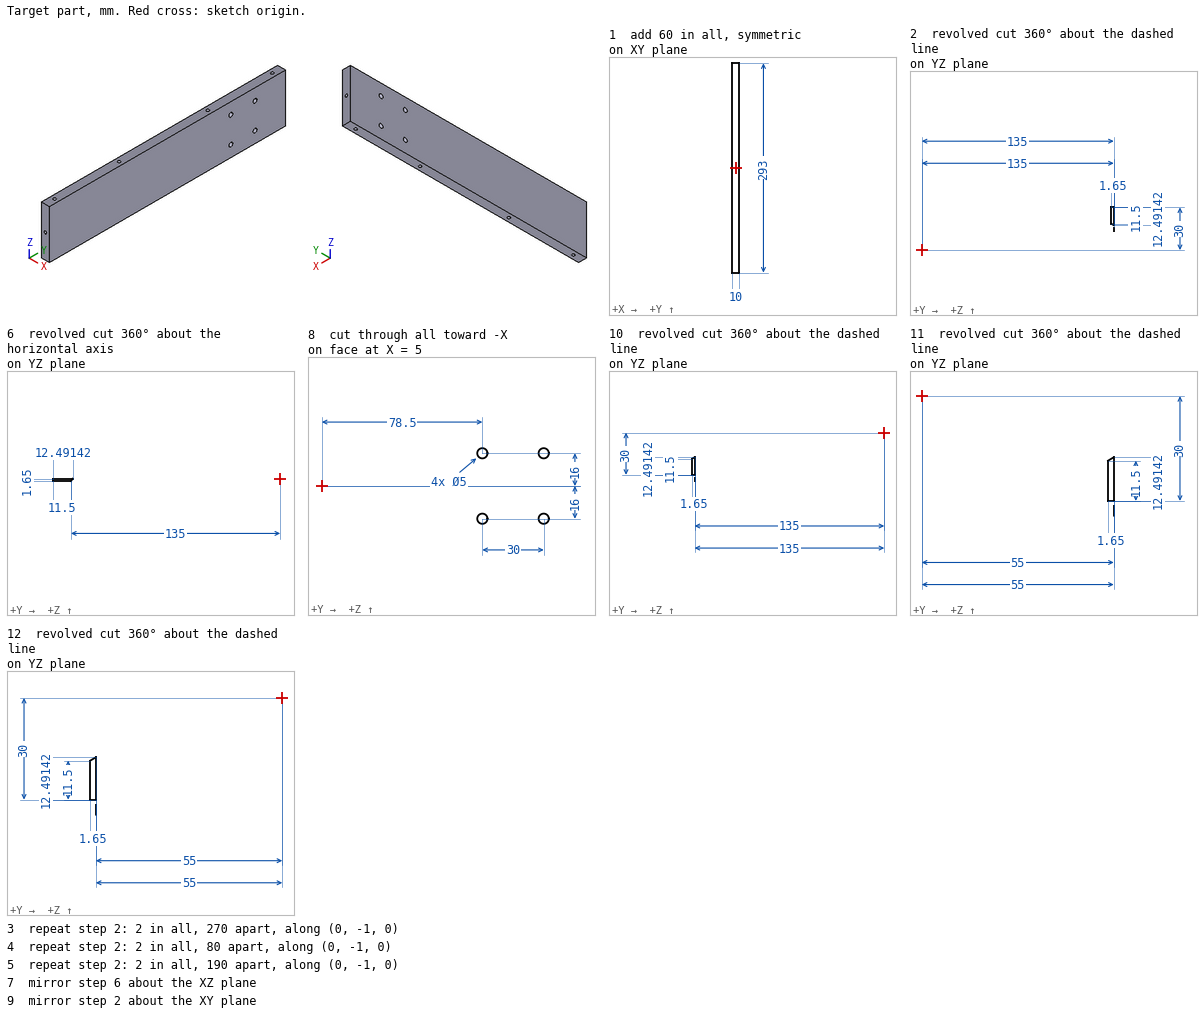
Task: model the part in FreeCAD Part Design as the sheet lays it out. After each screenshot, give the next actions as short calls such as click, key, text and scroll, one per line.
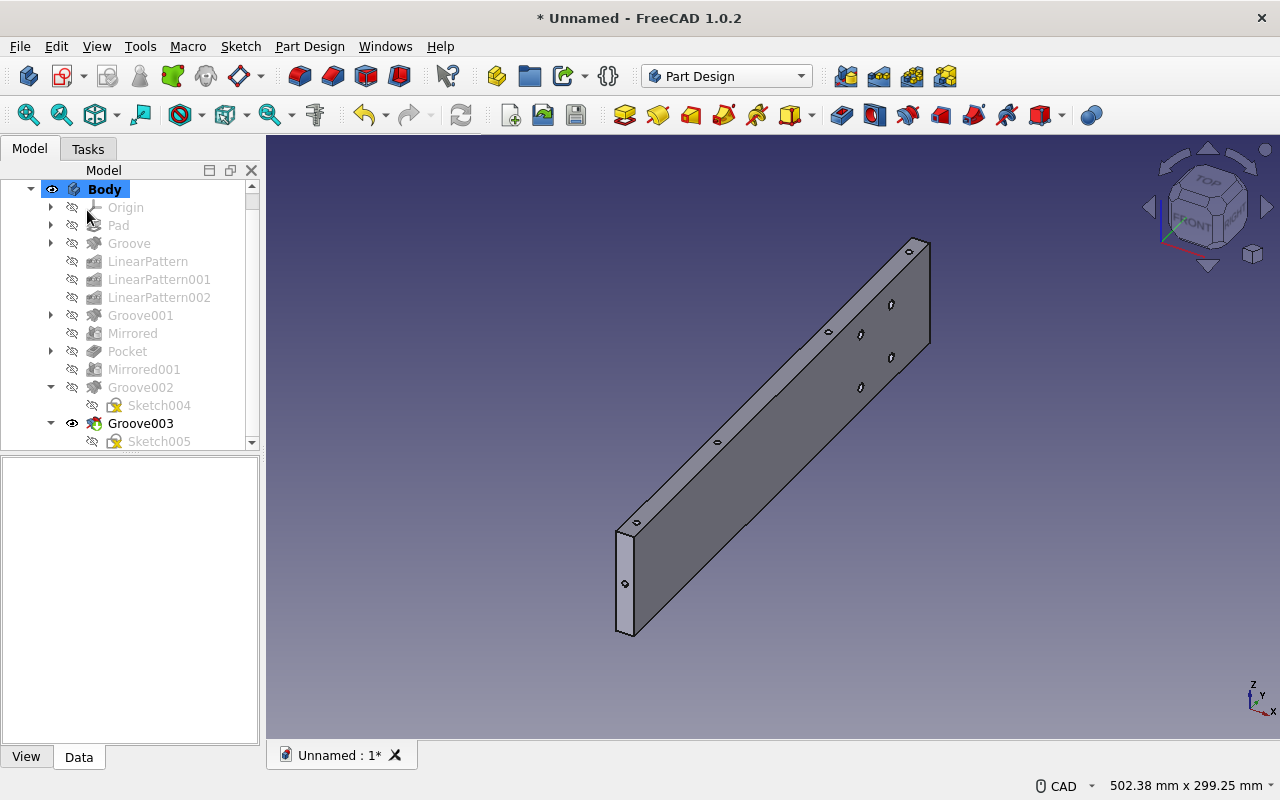
click(62, 76)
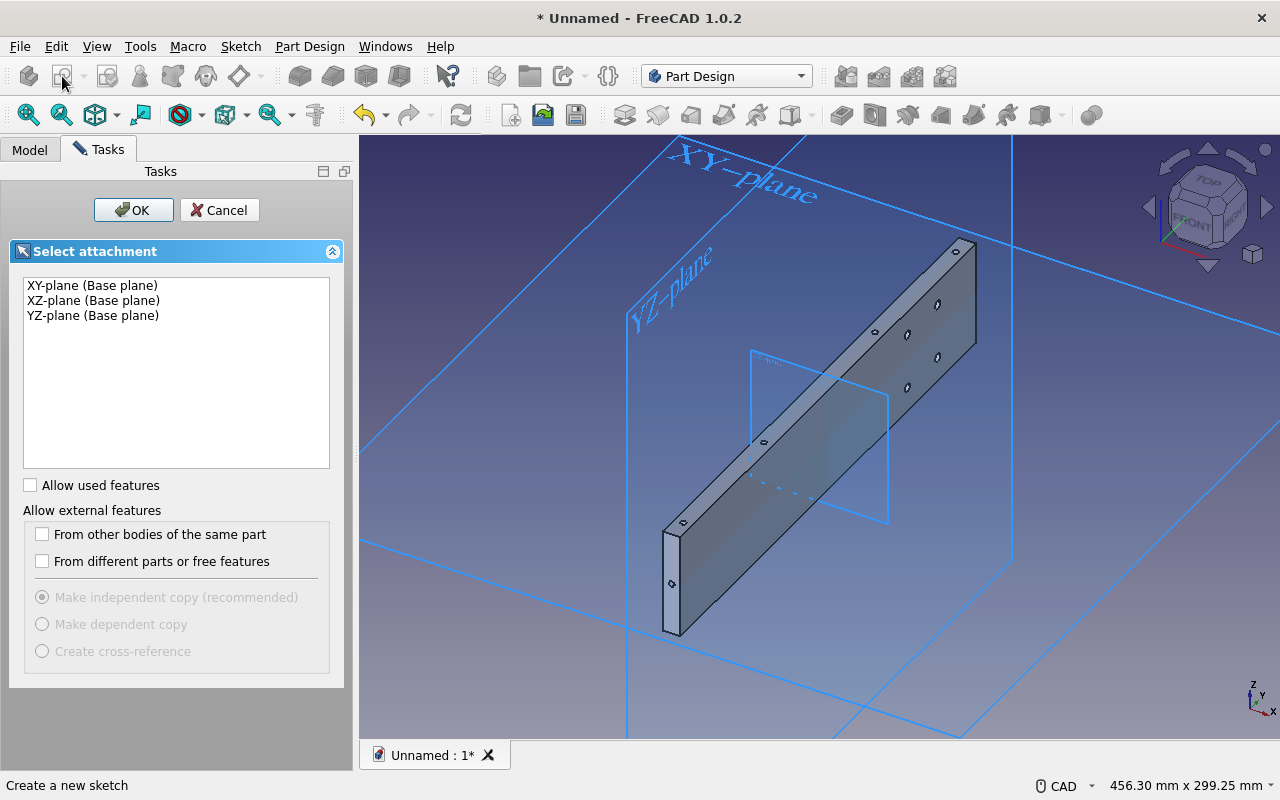
click(84, 316)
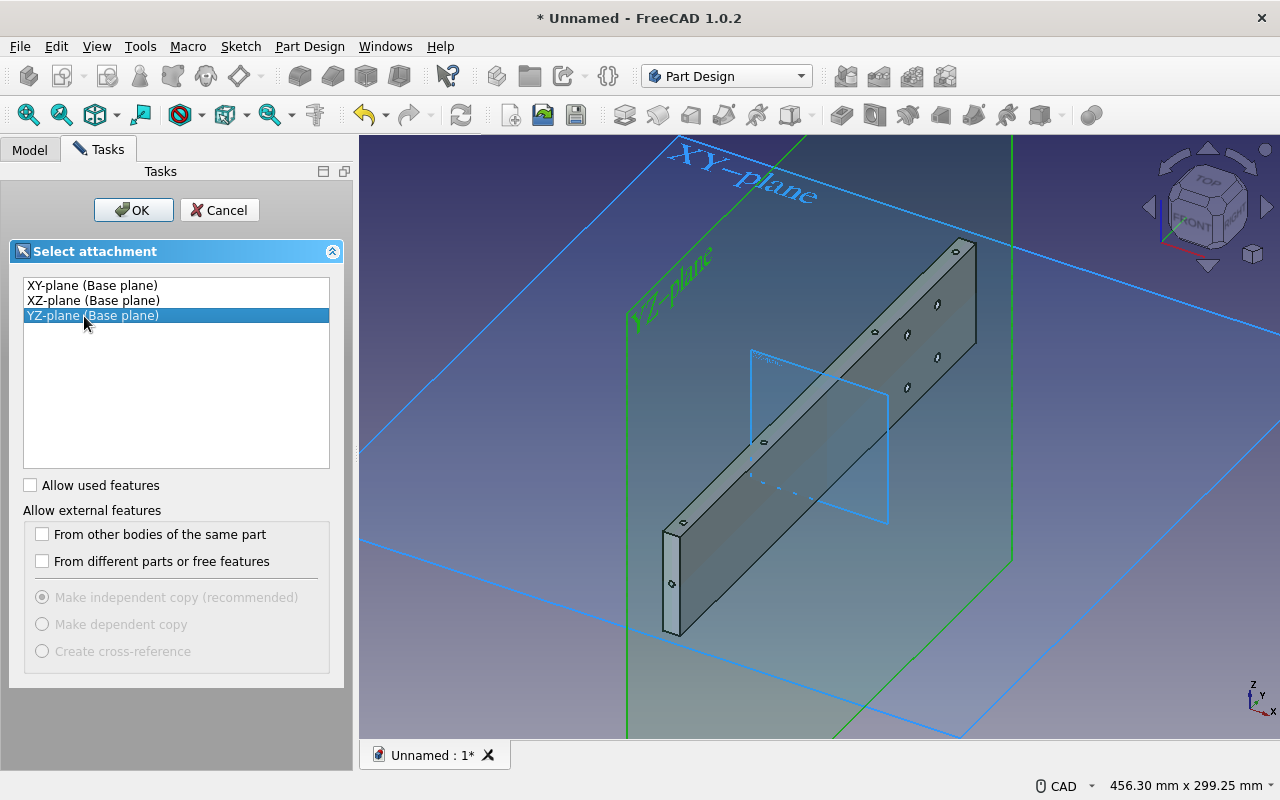
click(134, 210)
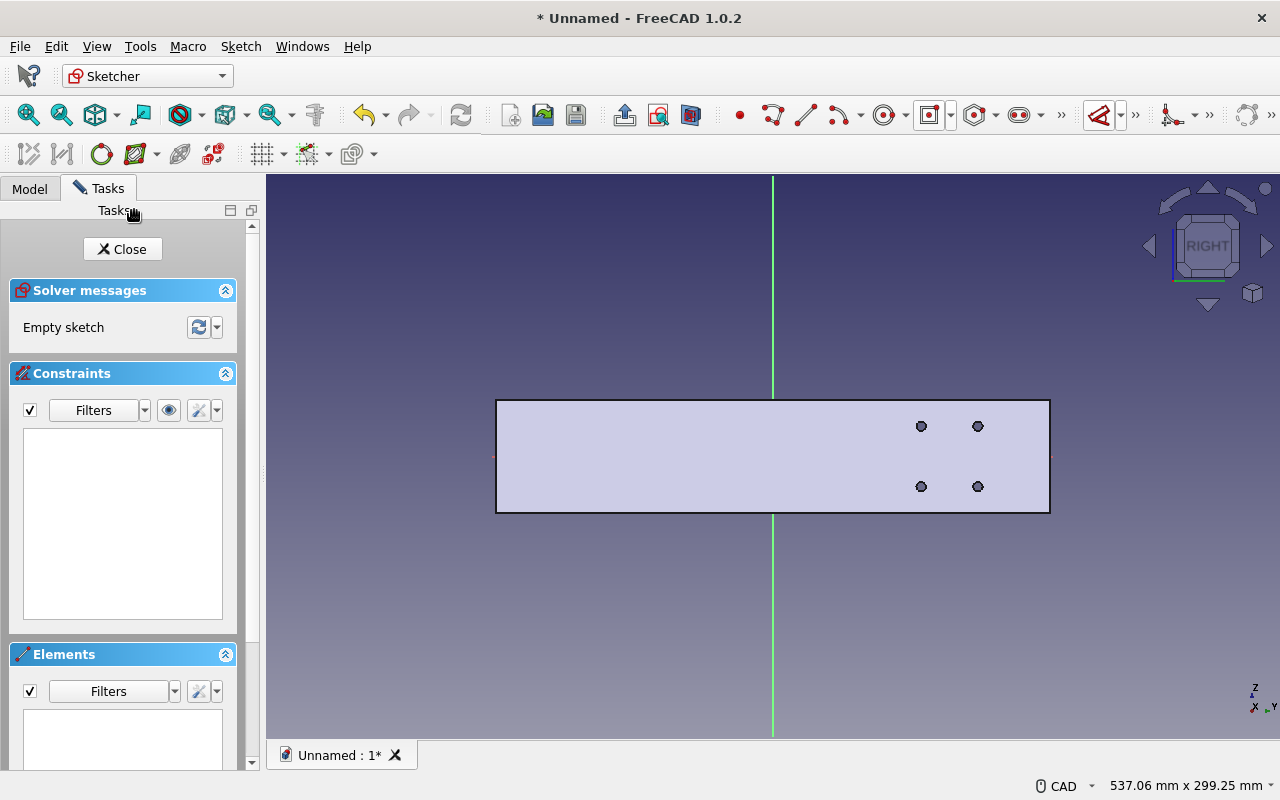
click(691, 116)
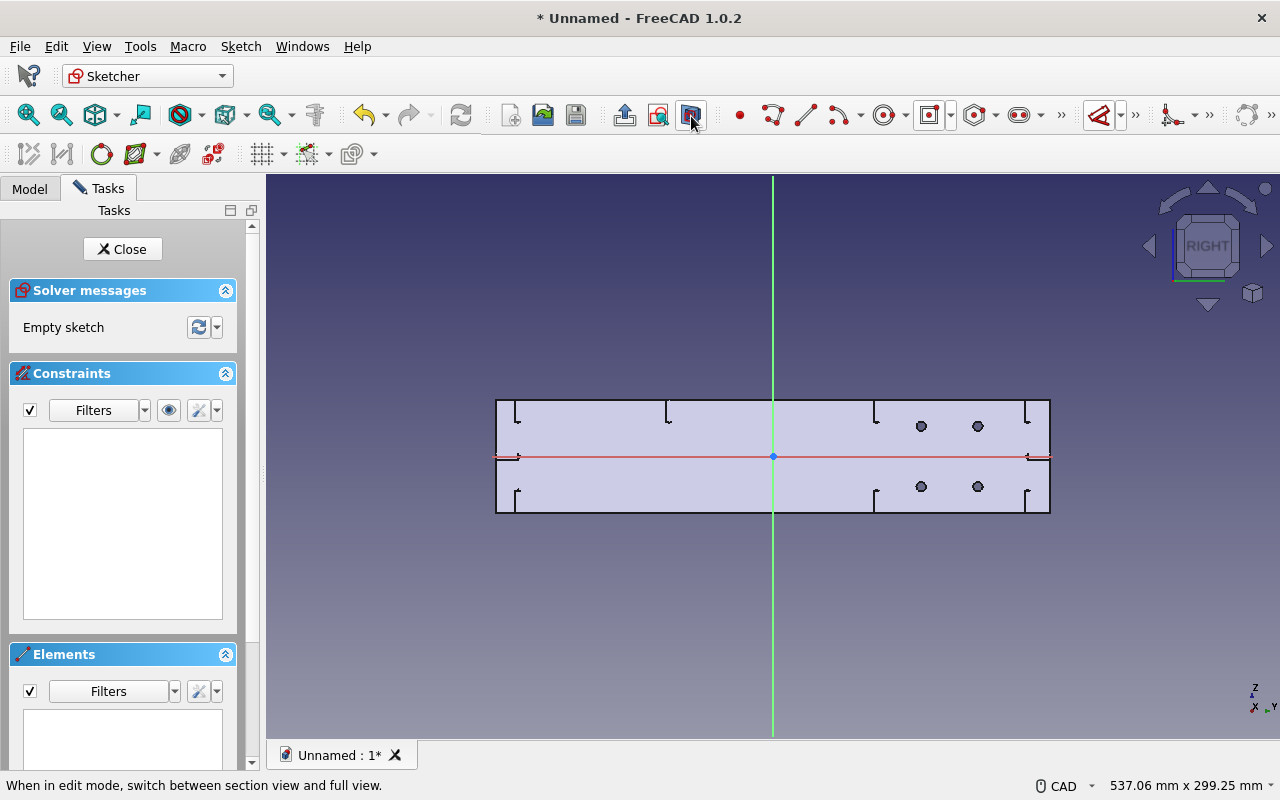
scroll(664, 511, up, 12)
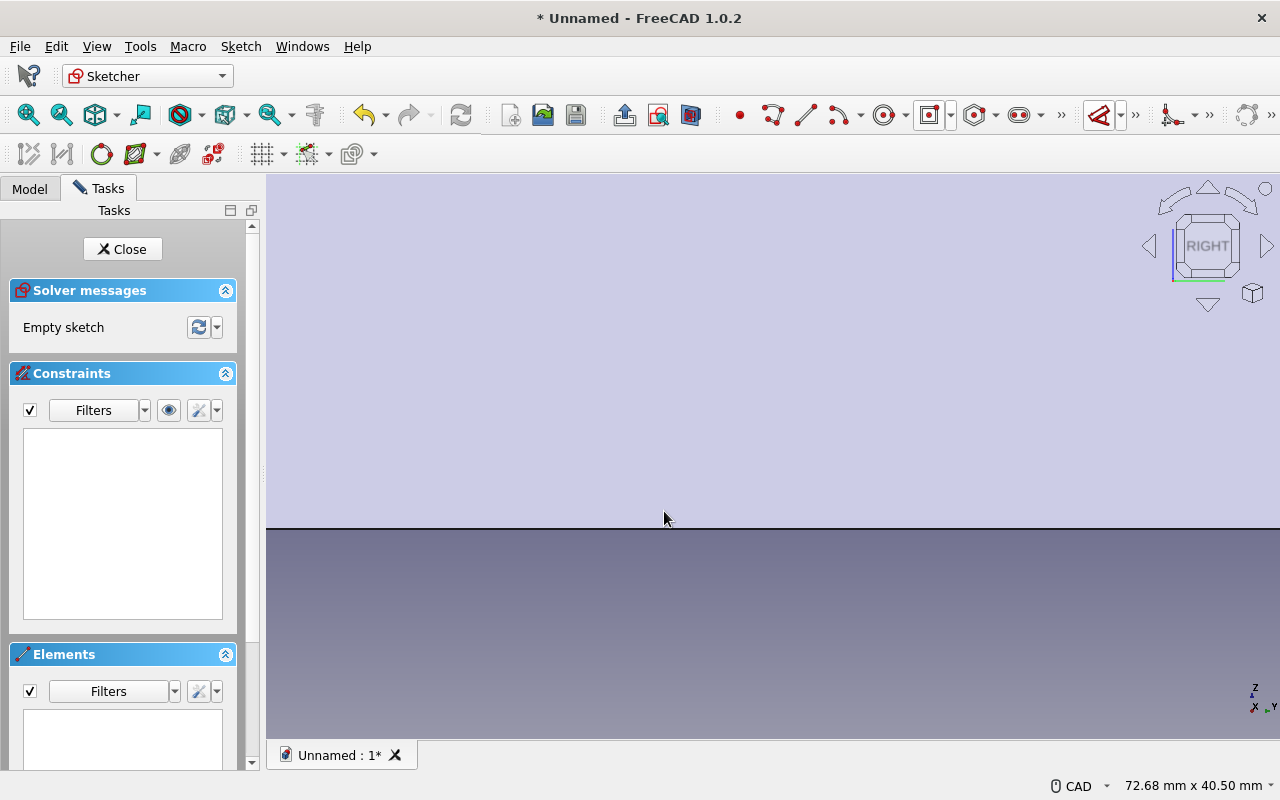
click(773, 116)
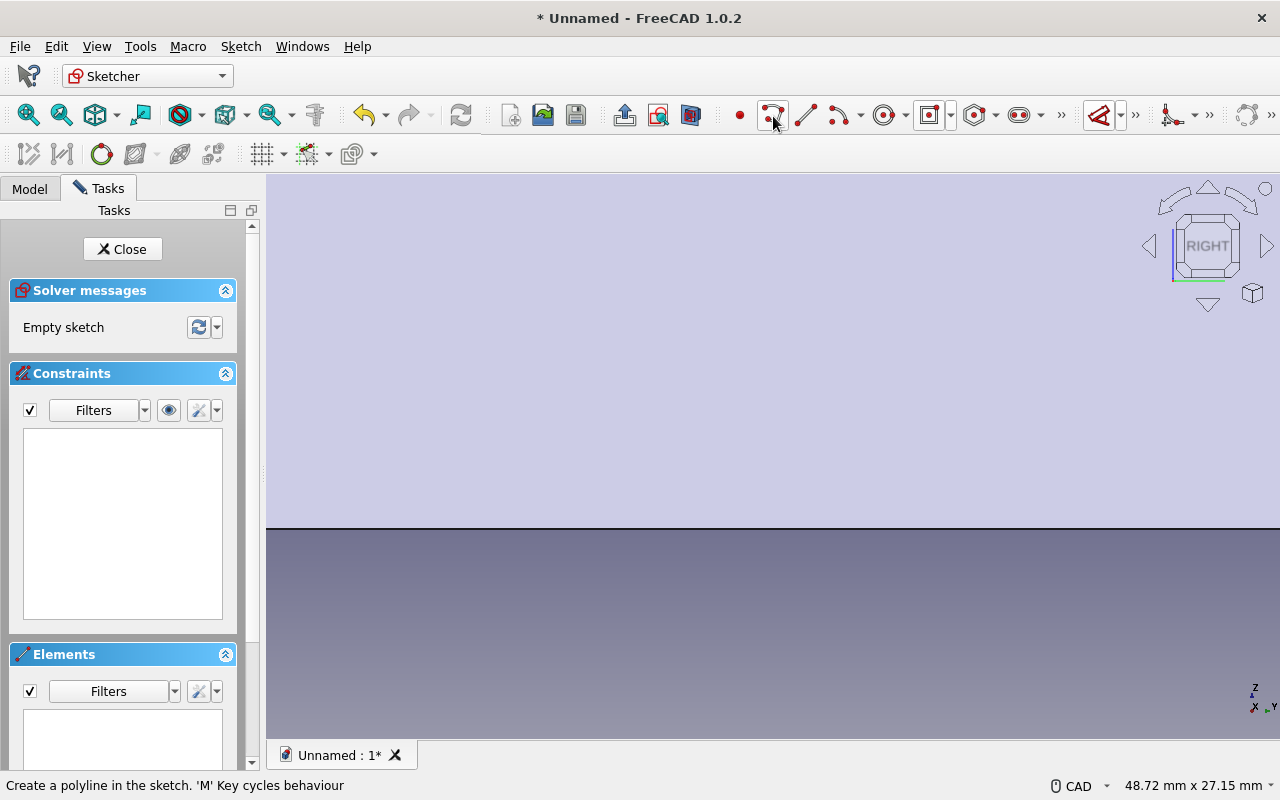
click(717, 269)
click(683, 289)
click(683, 529)
click(717, 529)
click(717, 270)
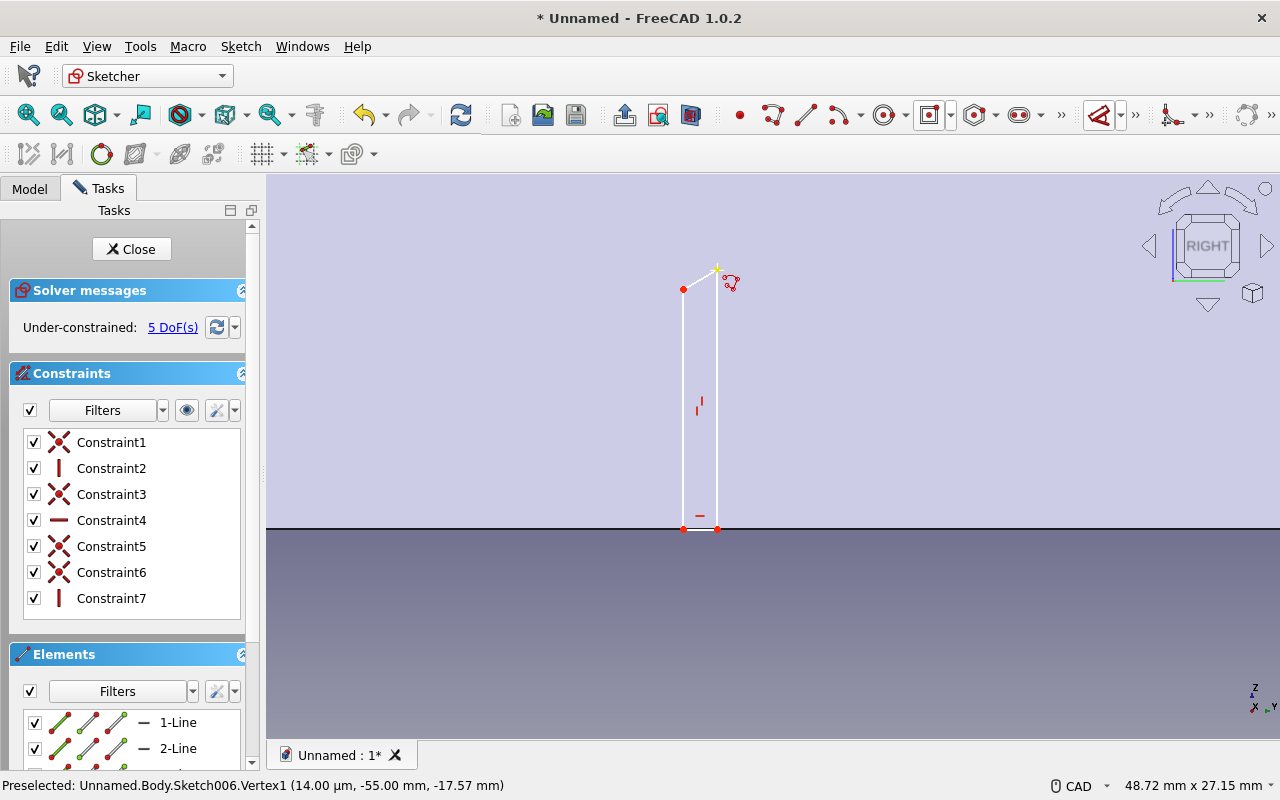
click(806, 116)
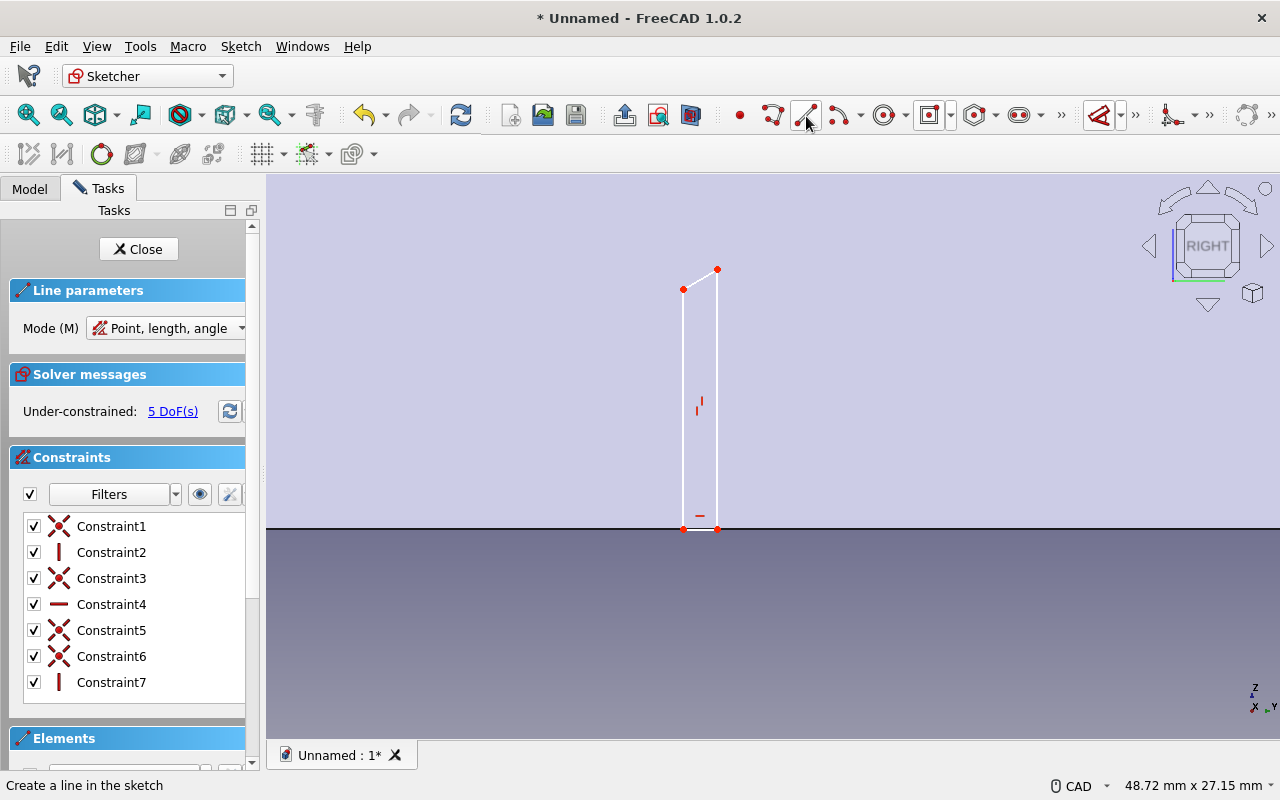
click(717, 555)
click(717, 633)
key(Escape)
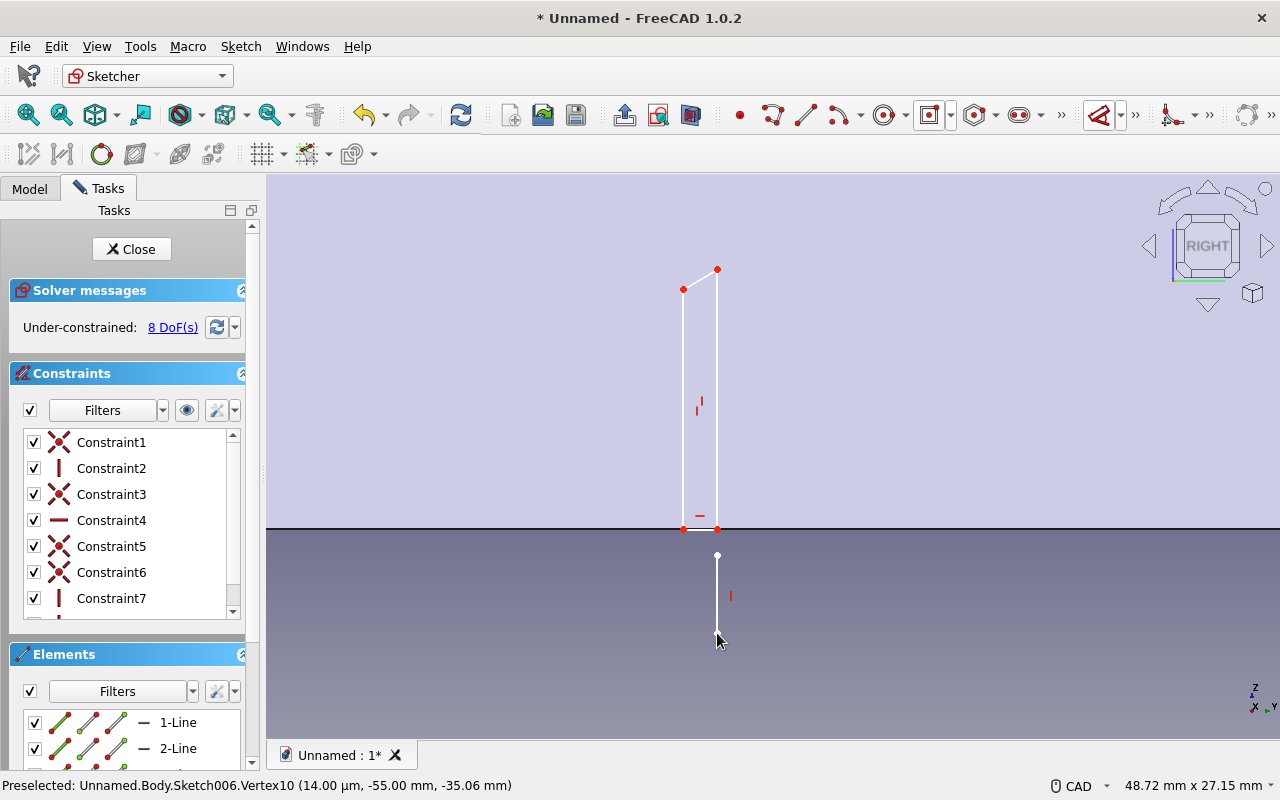
click(717, 579)